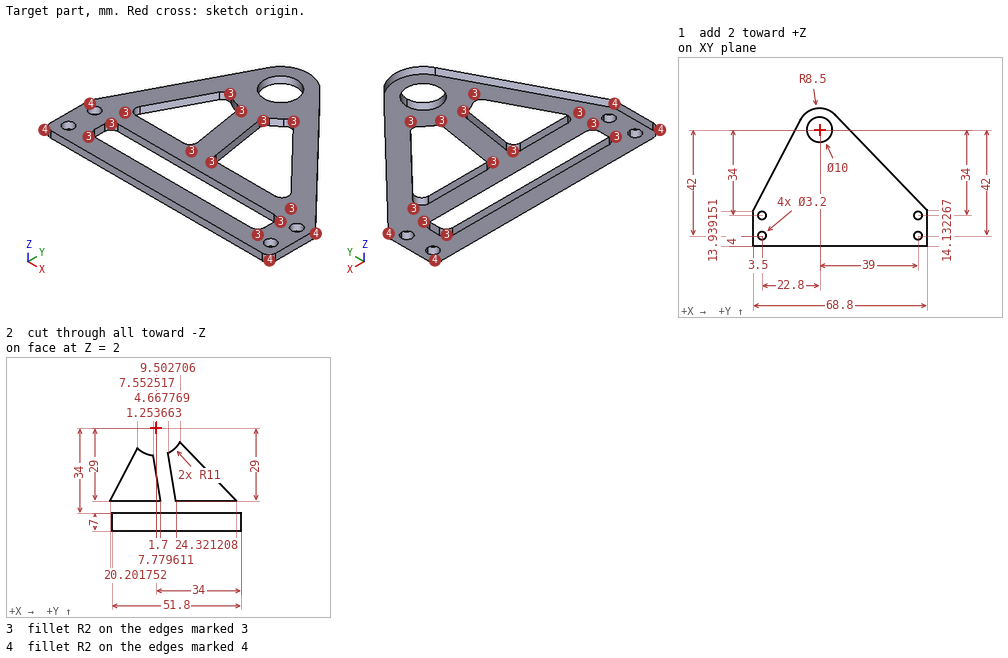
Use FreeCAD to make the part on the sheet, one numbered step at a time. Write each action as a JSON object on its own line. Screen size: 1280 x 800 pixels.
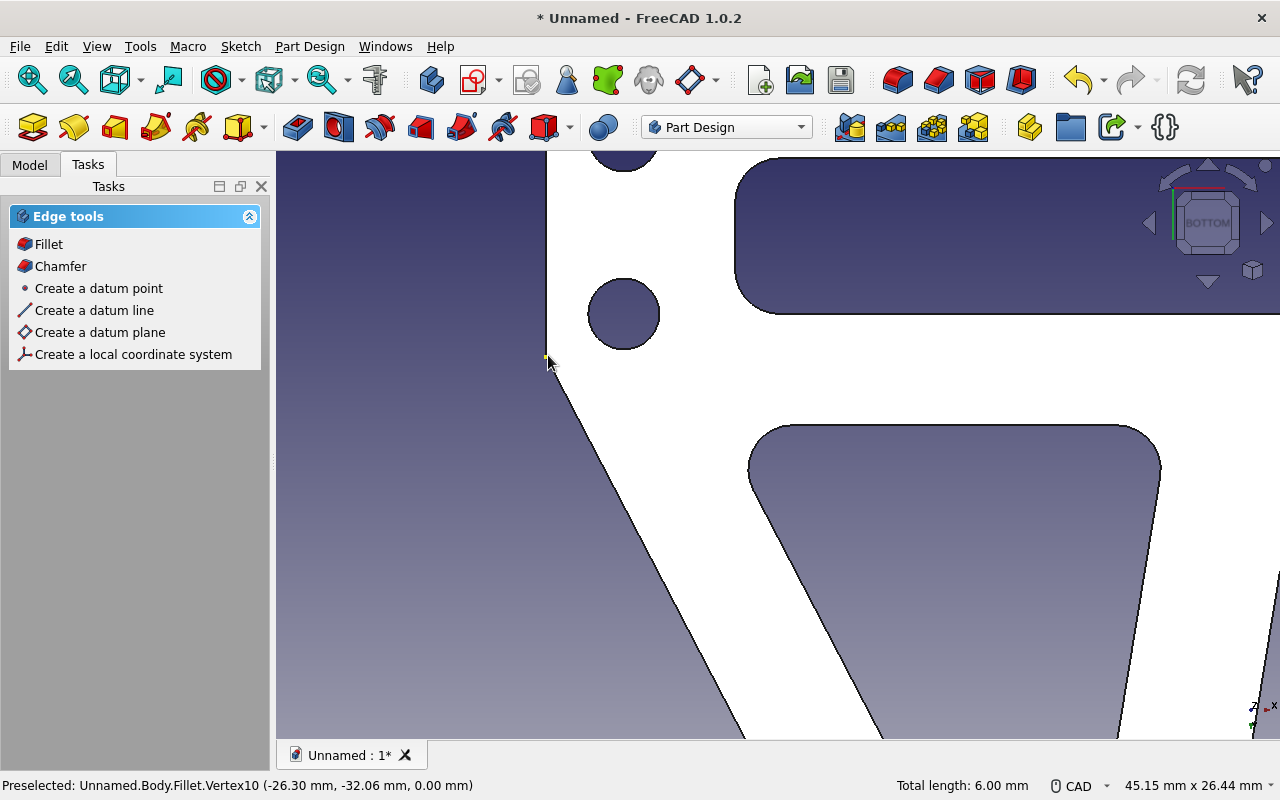
{"action": "key", "text": "v f"}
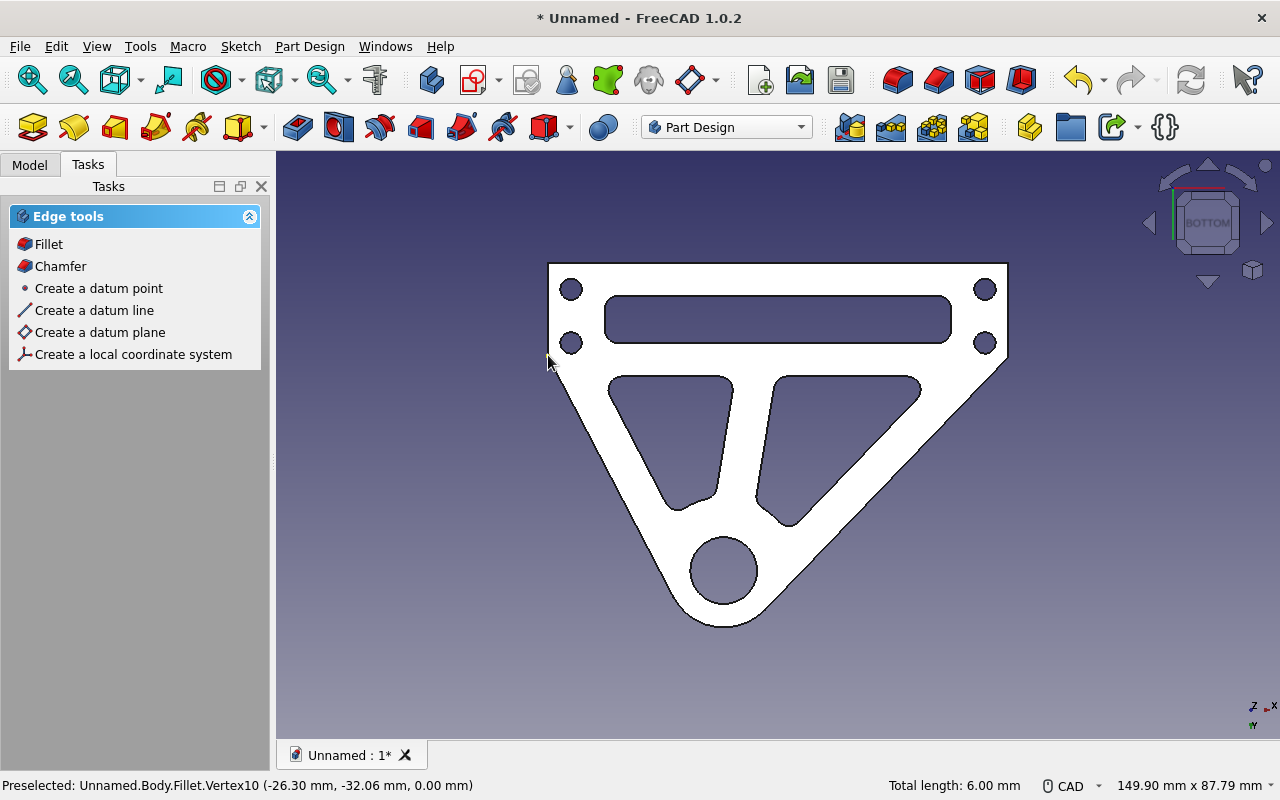
{"action": "key", "text": "4"}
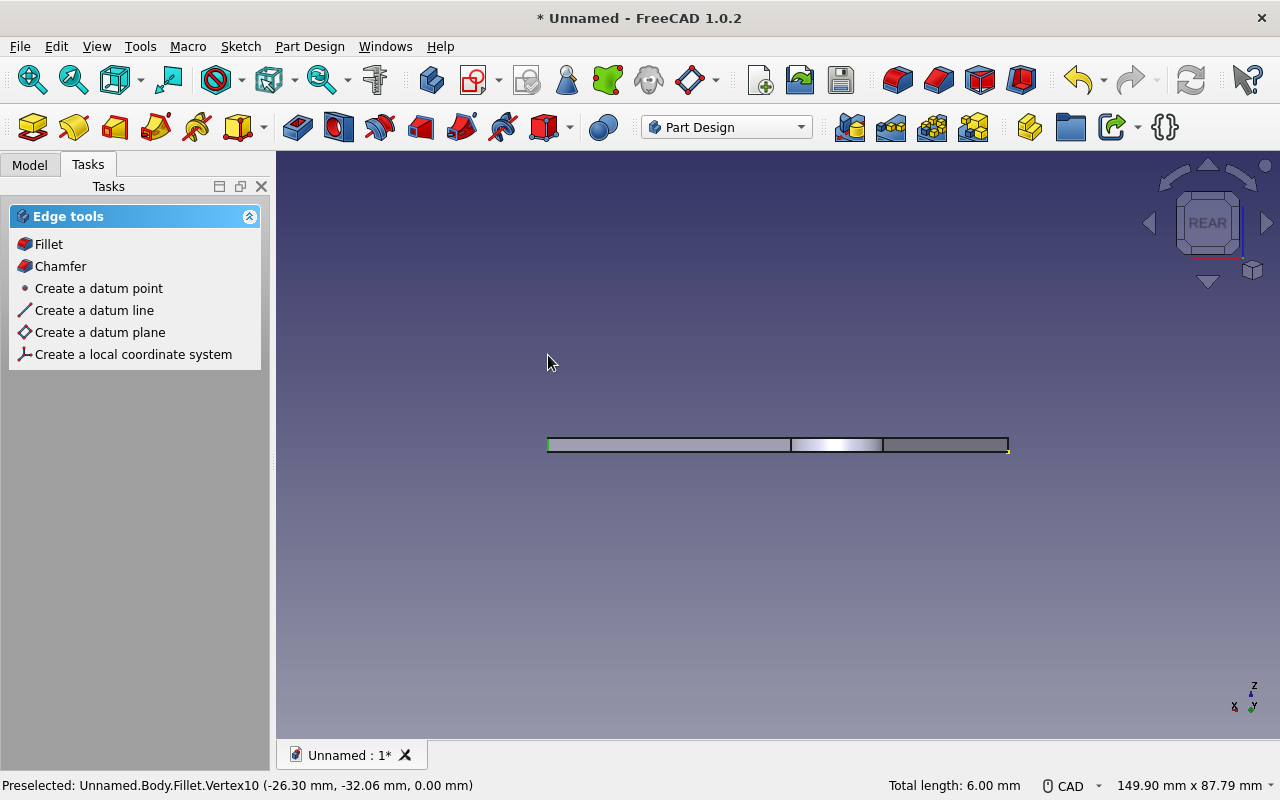
{"action": "scroll", "coordinate": [1008, 444], "scroll_direction": "up", "scroll_amount": 6}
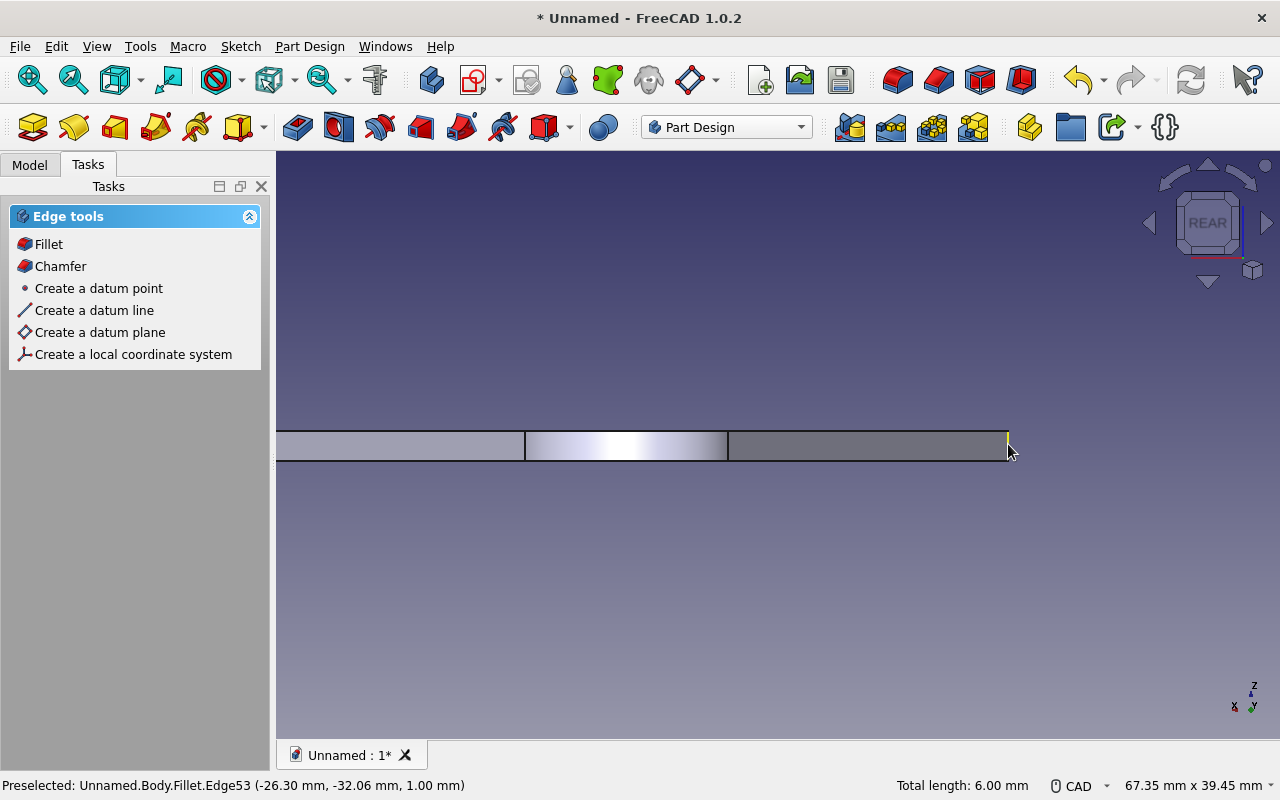
{"action": "key", "text": "v f"}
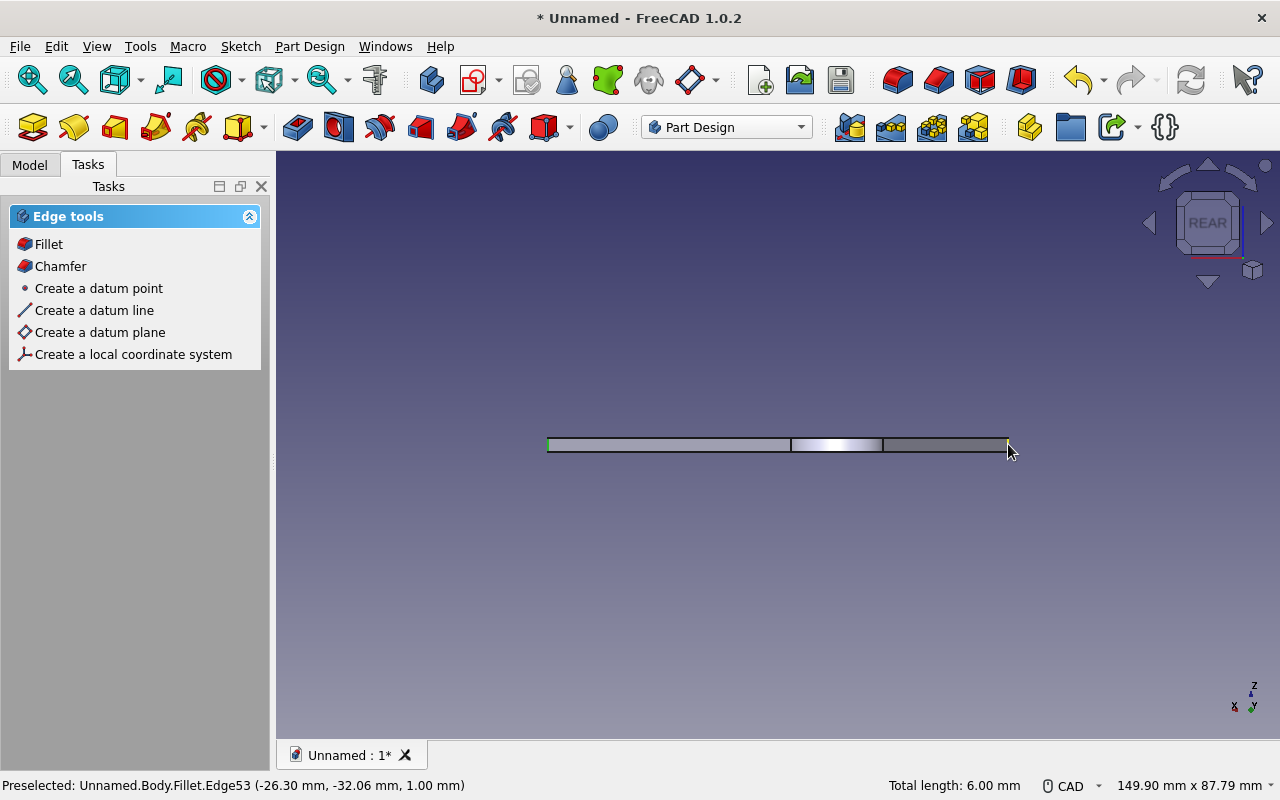
{"action": "key", "text": "6"}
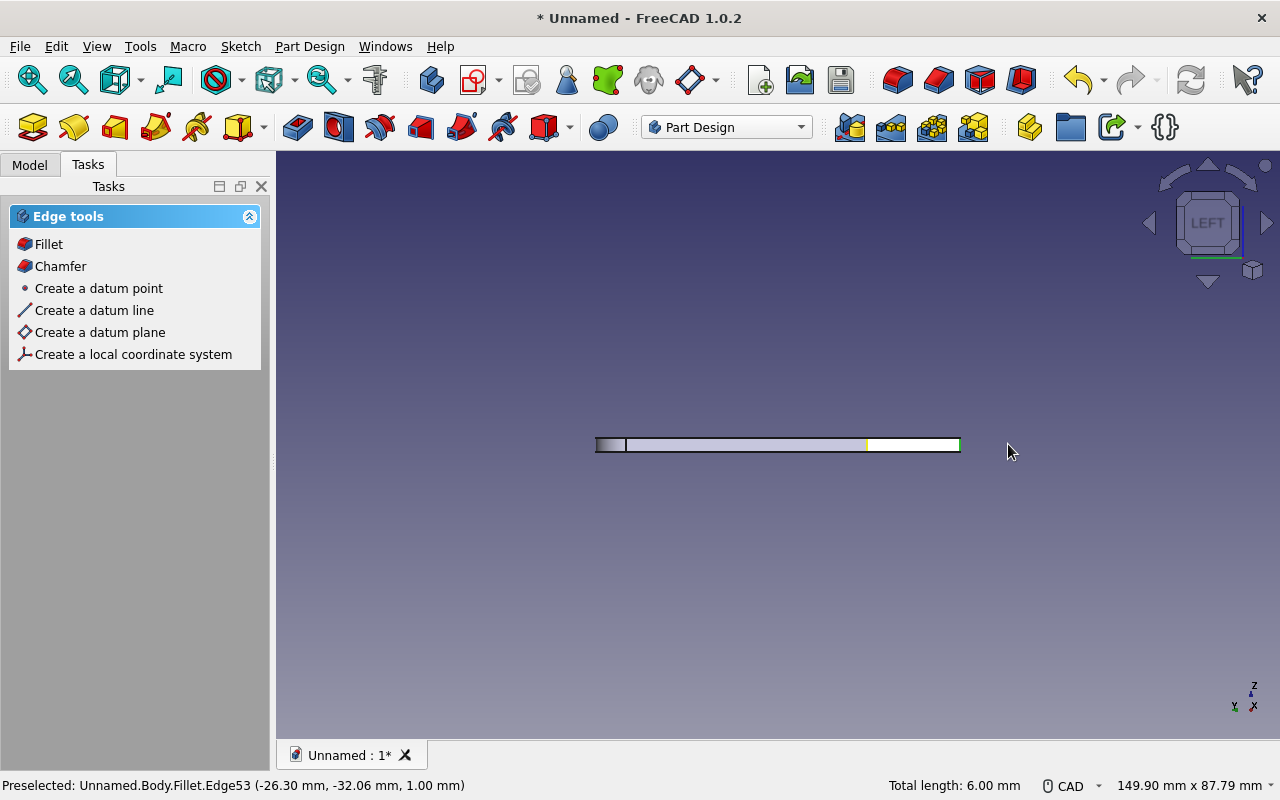
{"action": "left_click", "coordinate": [33, 80]}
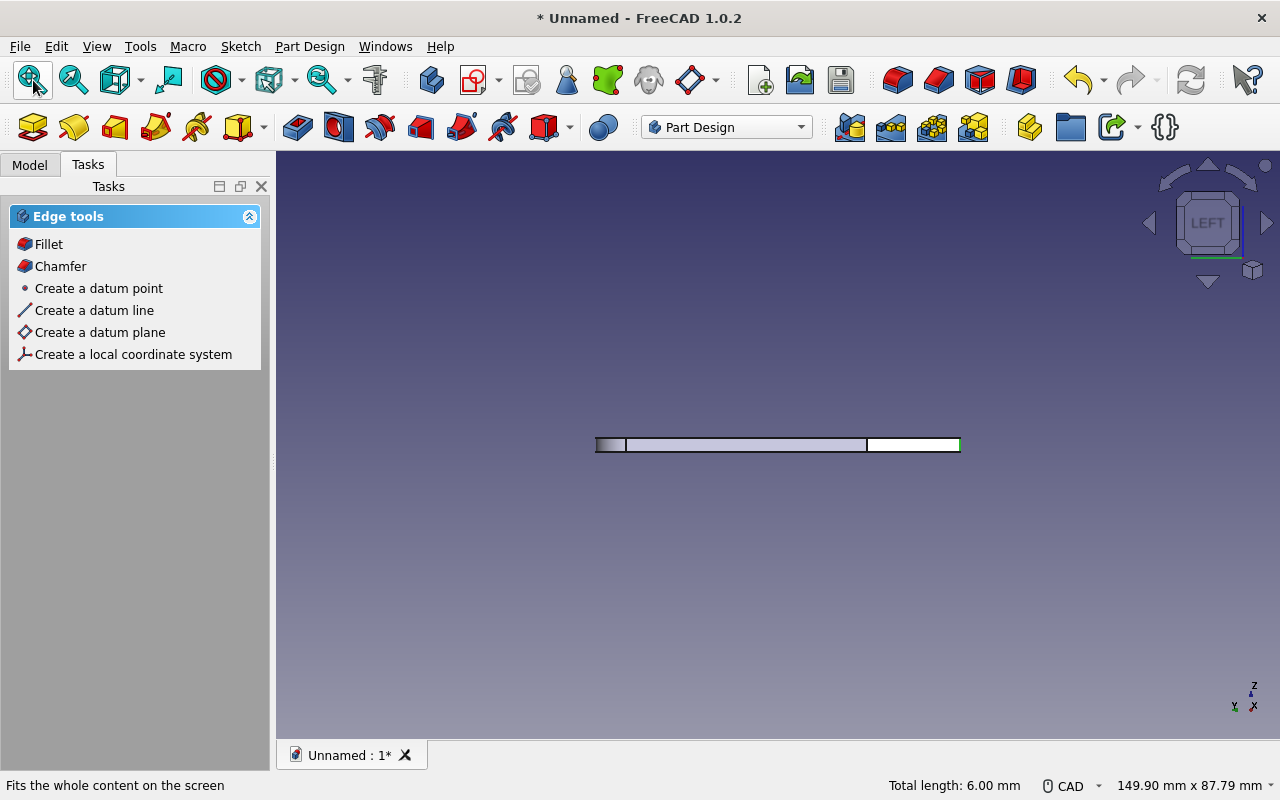
{"action": "left_click", "coordinate": [867, 444], "text": "ctrl"}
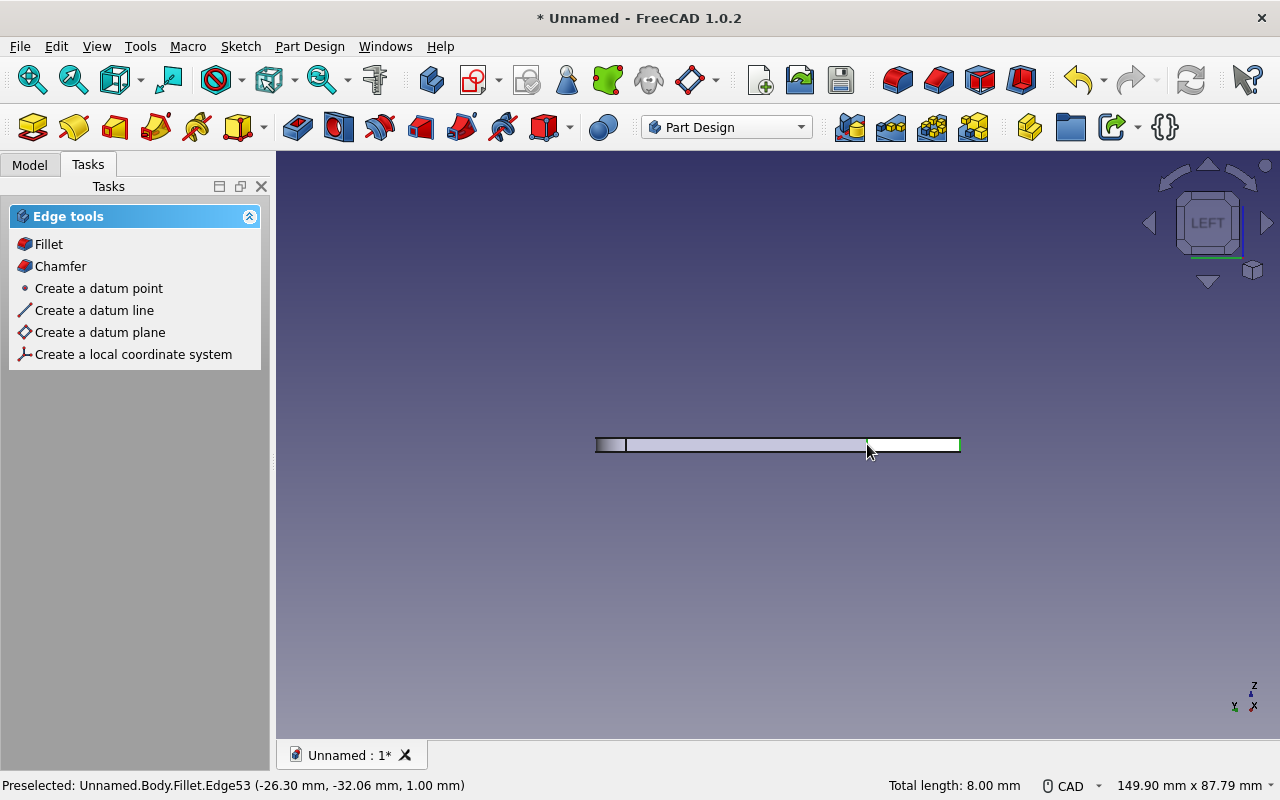
{"action": "left_click", "coordinate": [898, 80]}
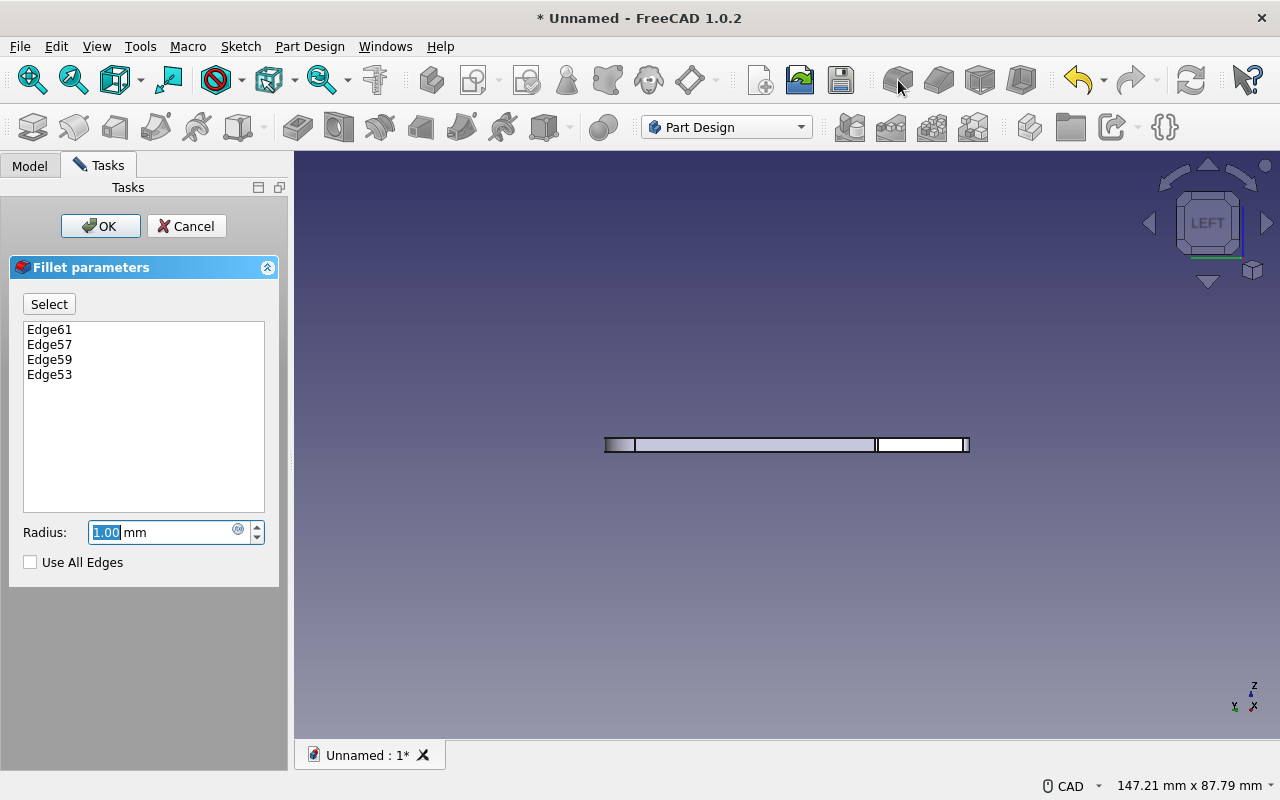
{"action": "type", "text": "2"}
{"action": "key", "text": "Tab"}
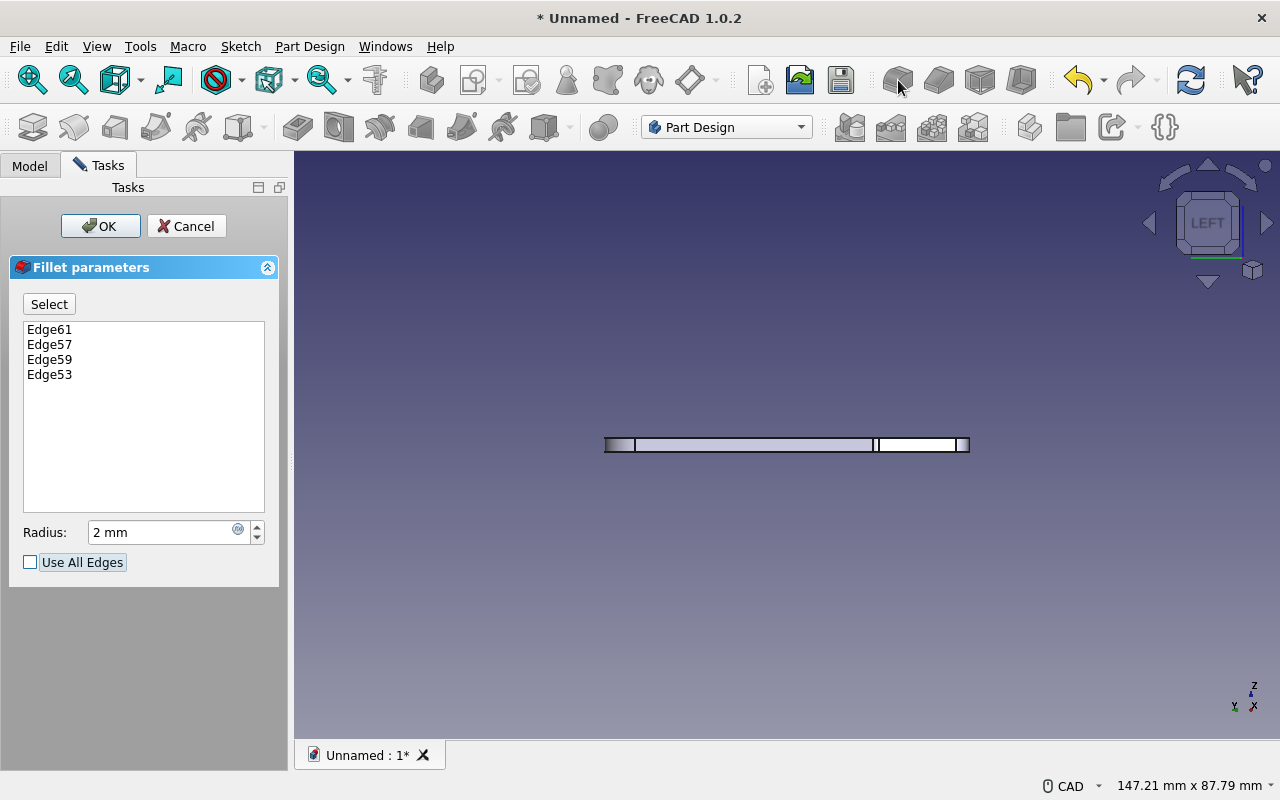
{"action": "left_click", "coordinate": [101, 226]}